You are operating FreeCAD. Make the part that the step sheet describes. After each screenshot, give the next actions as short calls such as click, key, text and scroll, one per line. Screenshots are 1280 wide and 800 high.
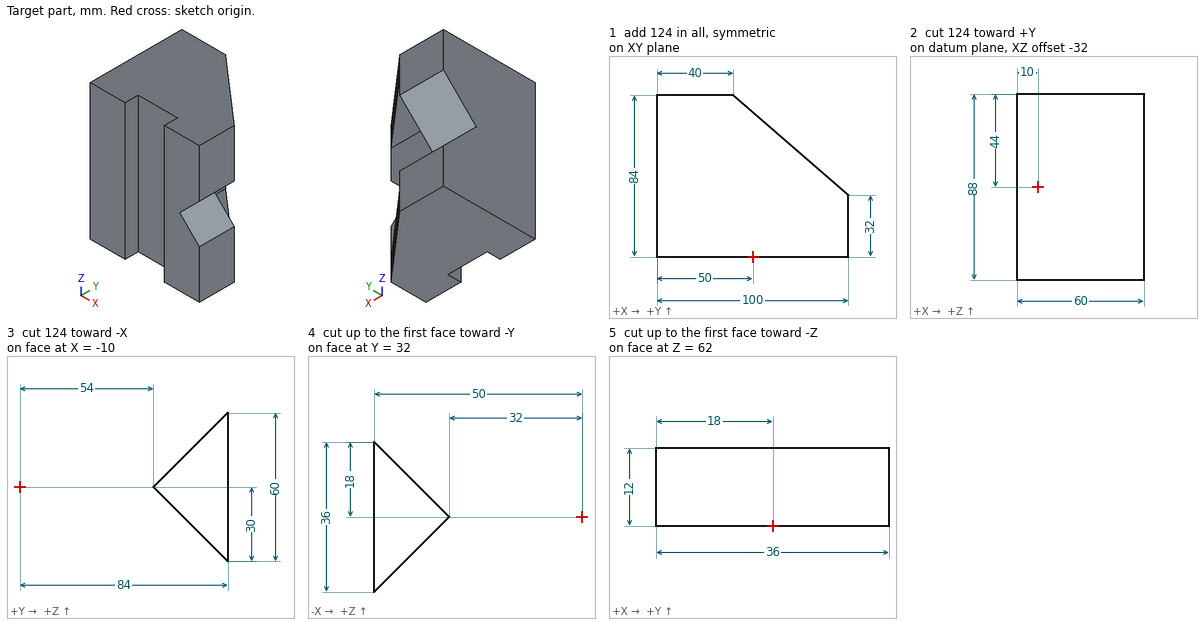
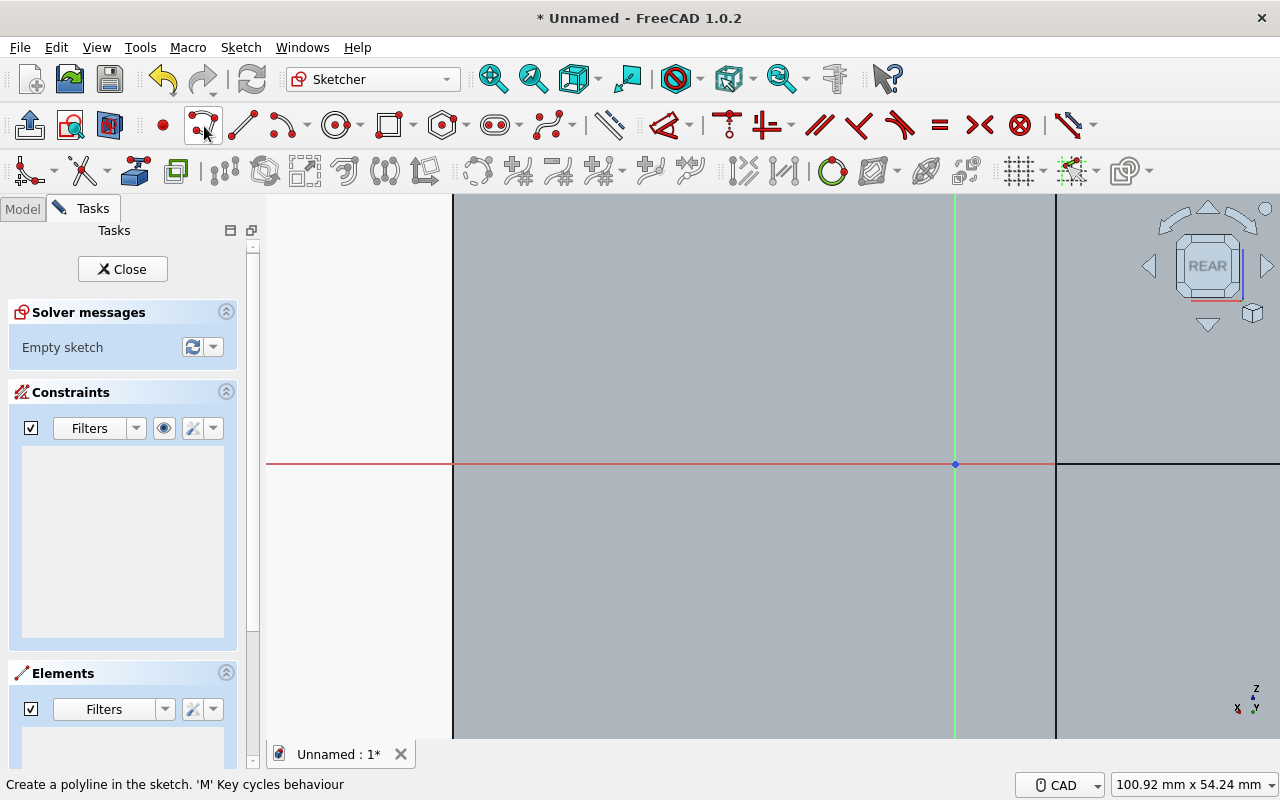
click(634, 464)
click(453, 283)
click(453, 645)
click(634, 464)
key(Escape)
key(Escape)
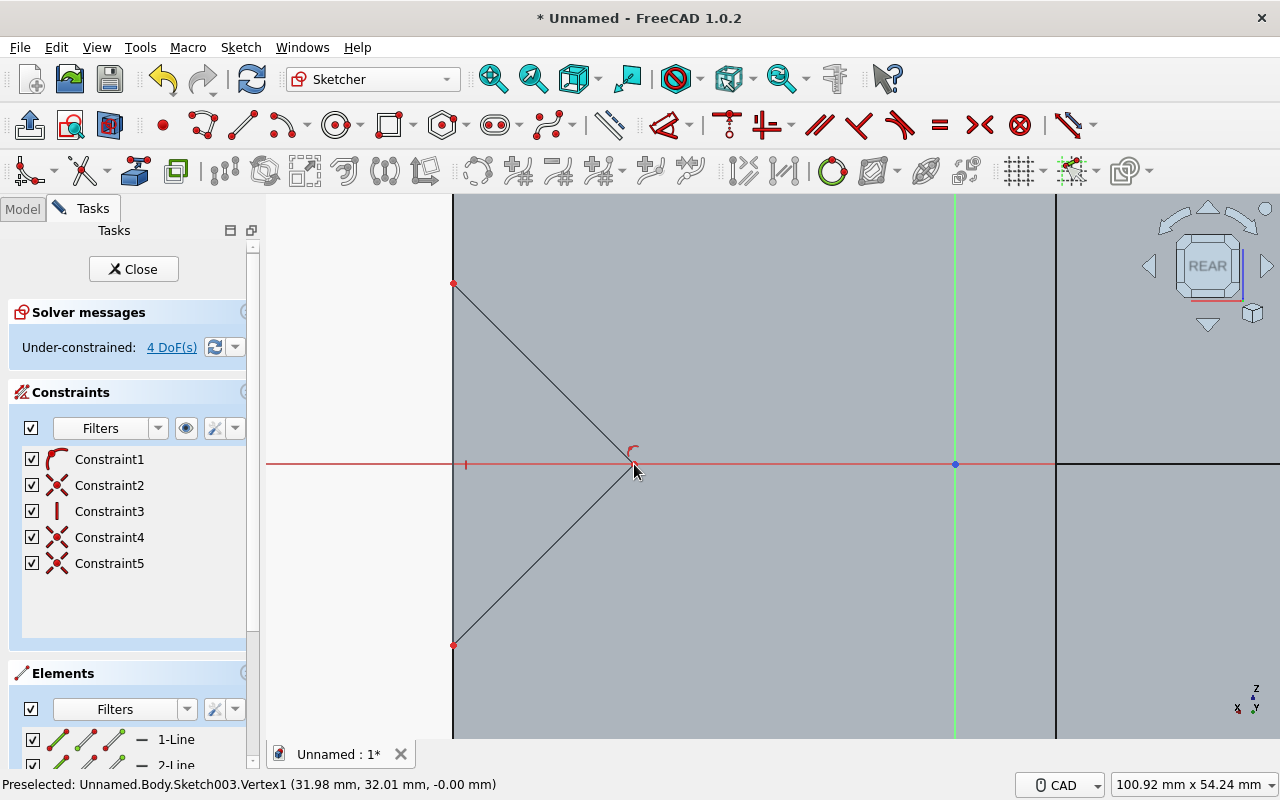
click(664, 126)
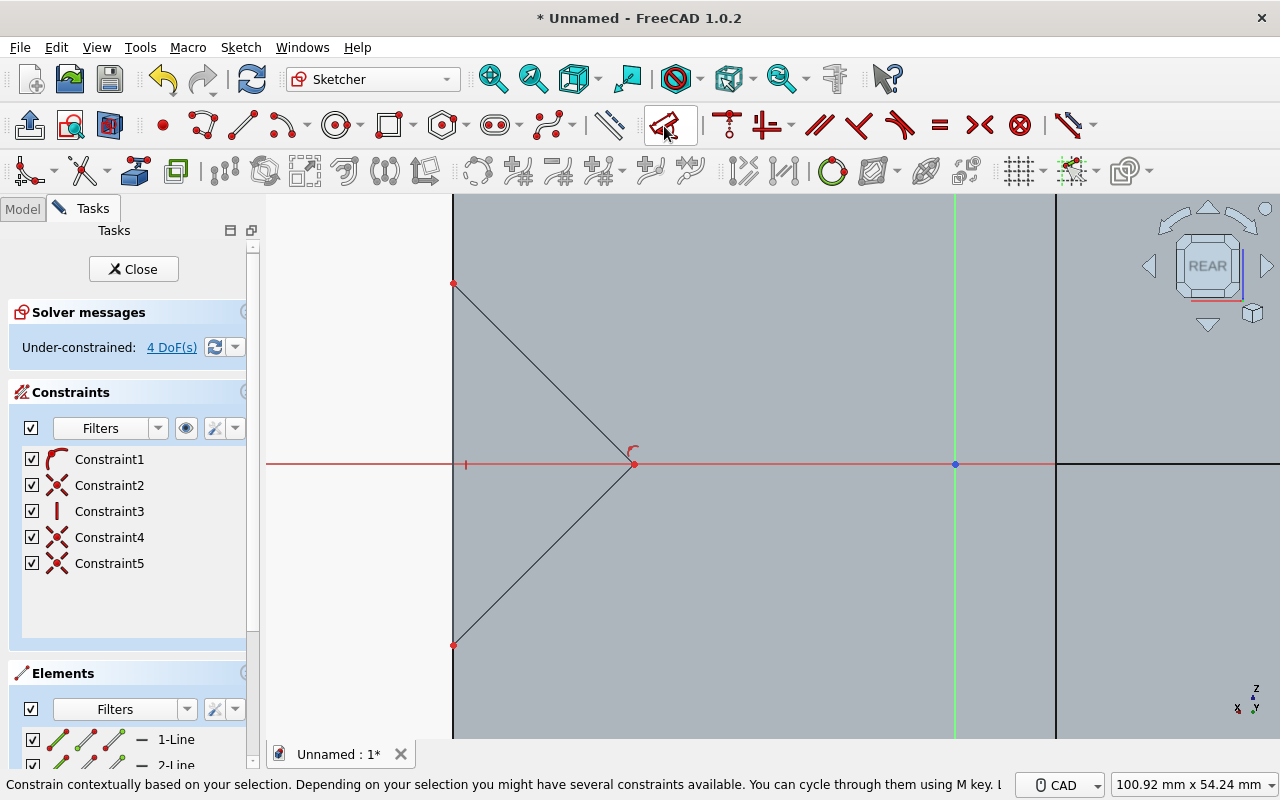
click(453, 393)
click(419, 382)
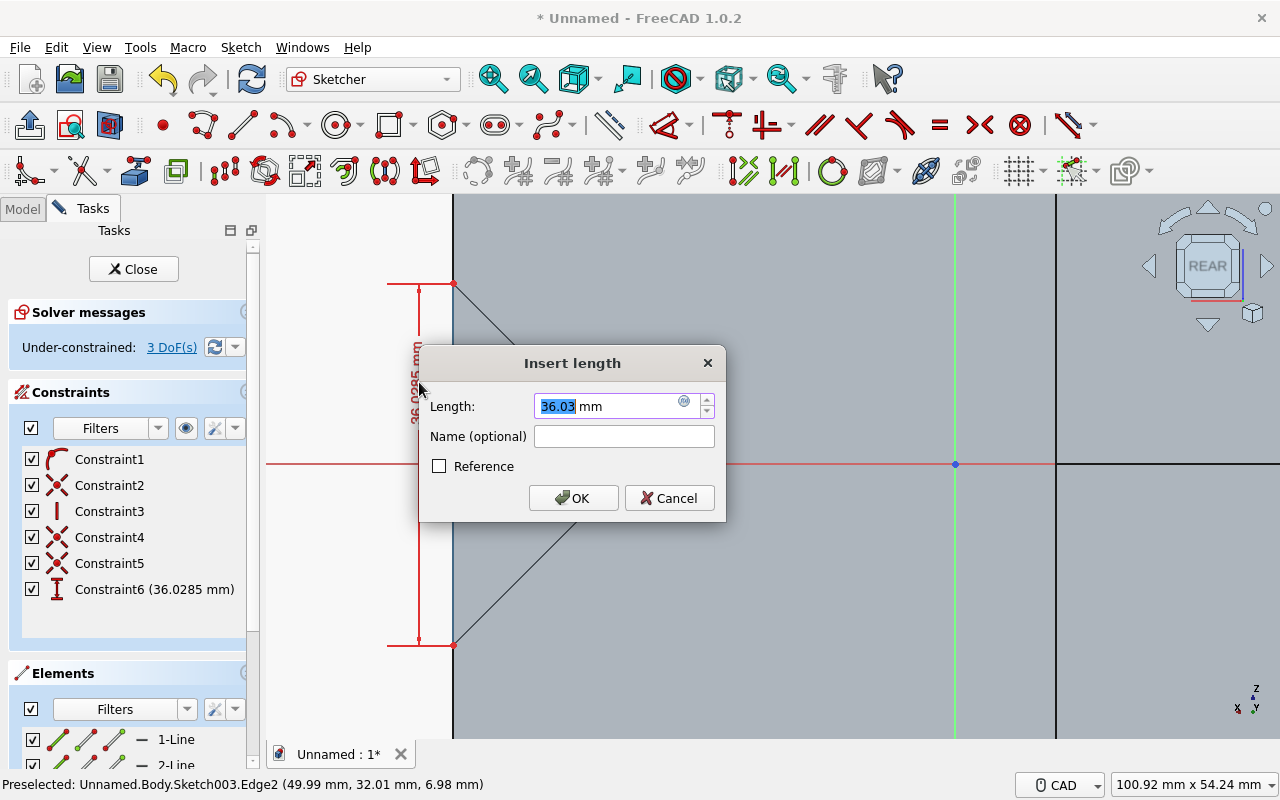
text(36)
key(Return)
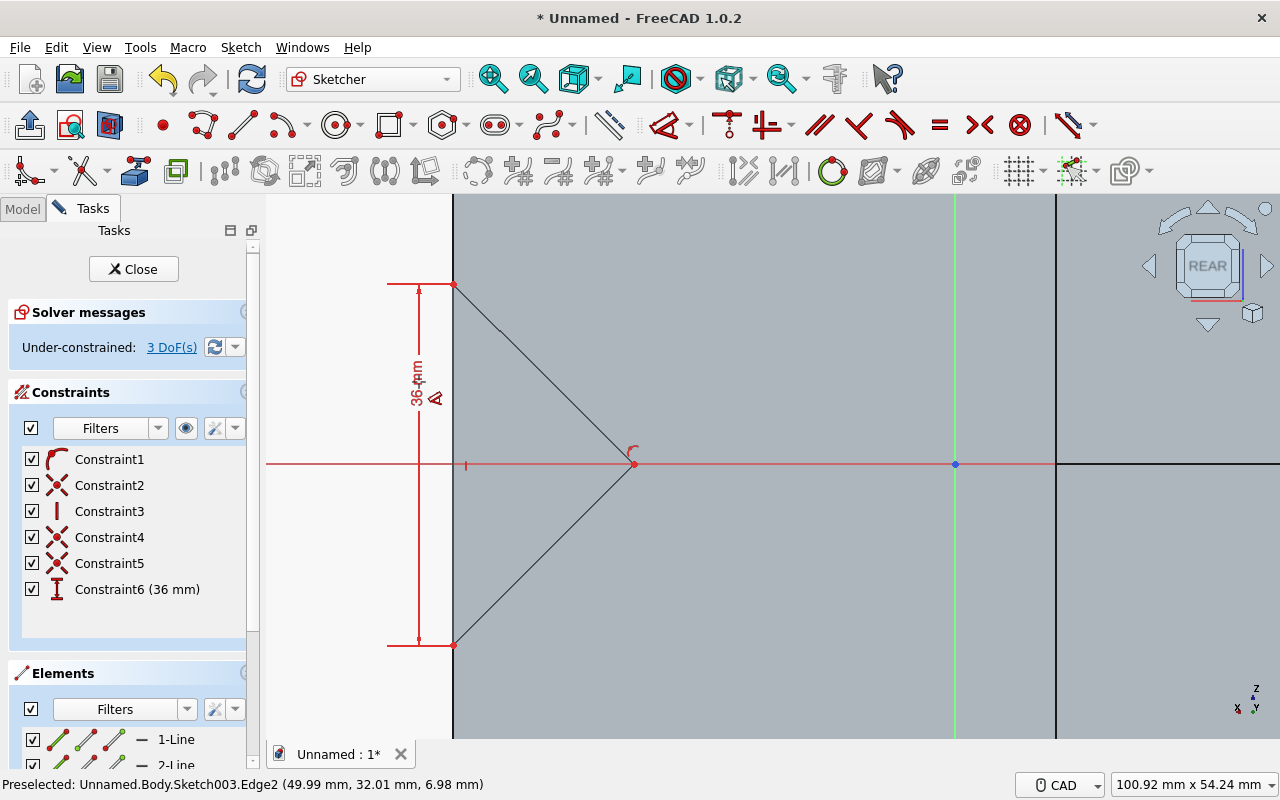
click(634, 464)
click(795, 498)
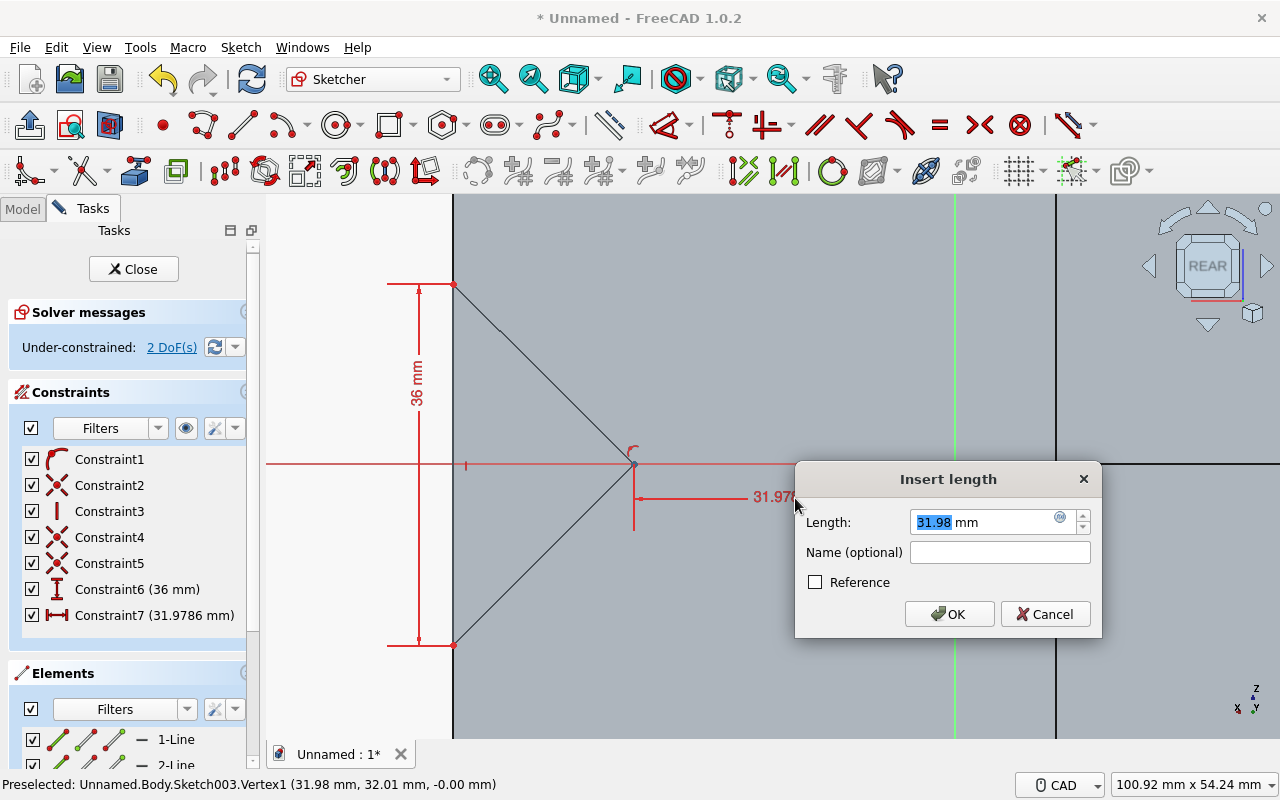
text(32)
key(Return)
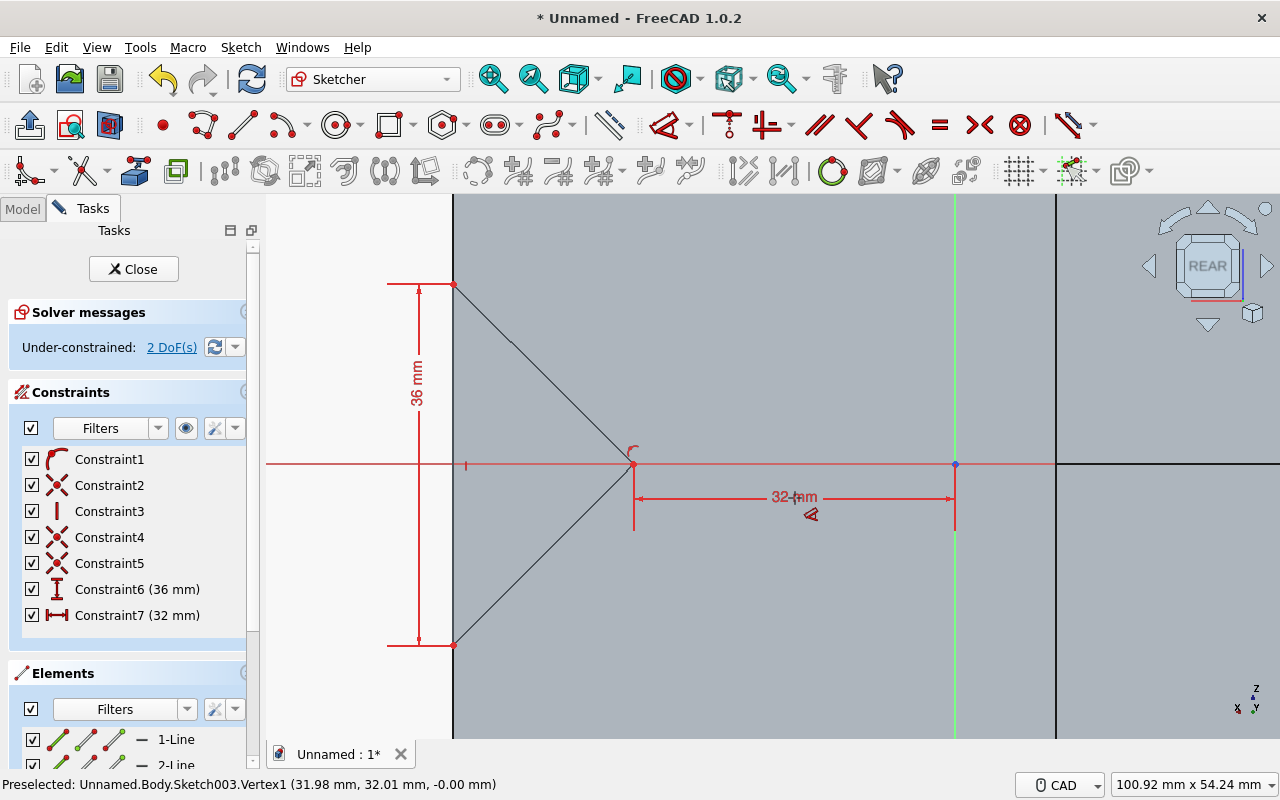
click(453, 284)
click(704, 250)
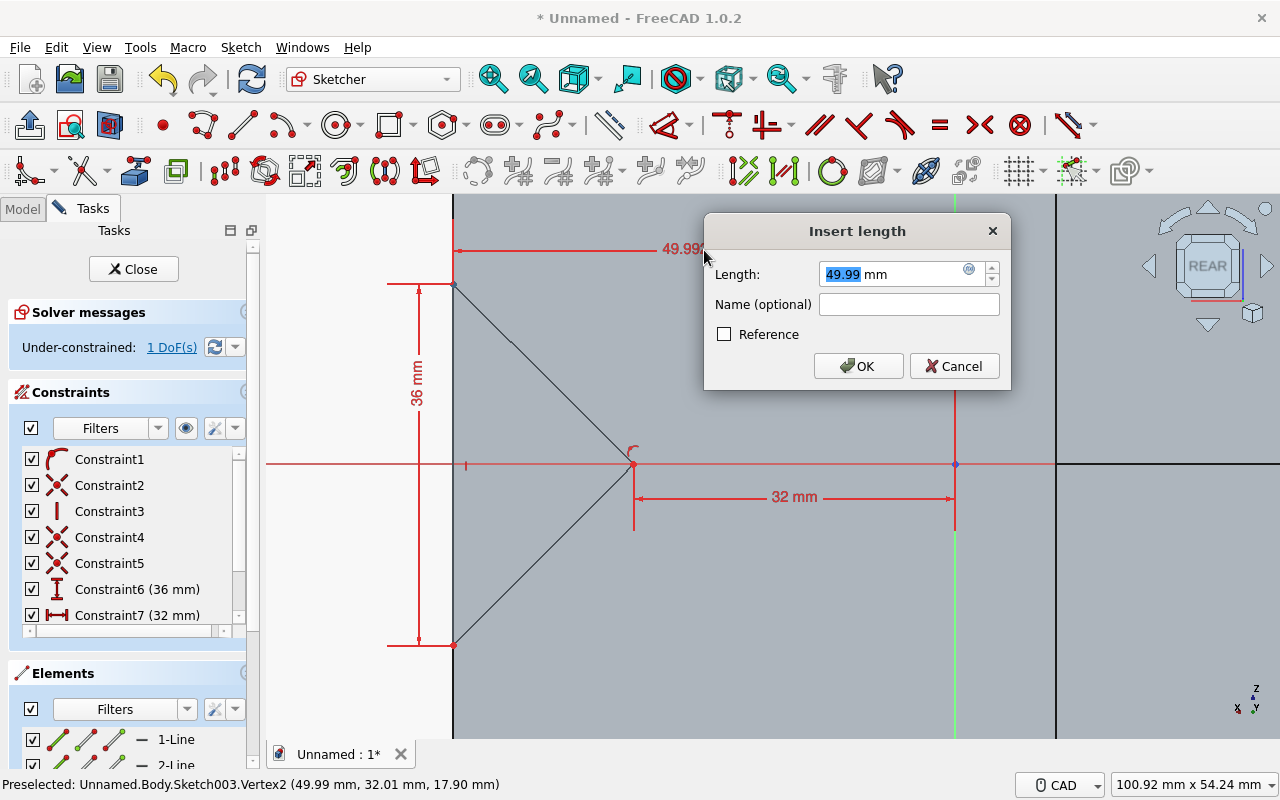
text(50)
key(Return)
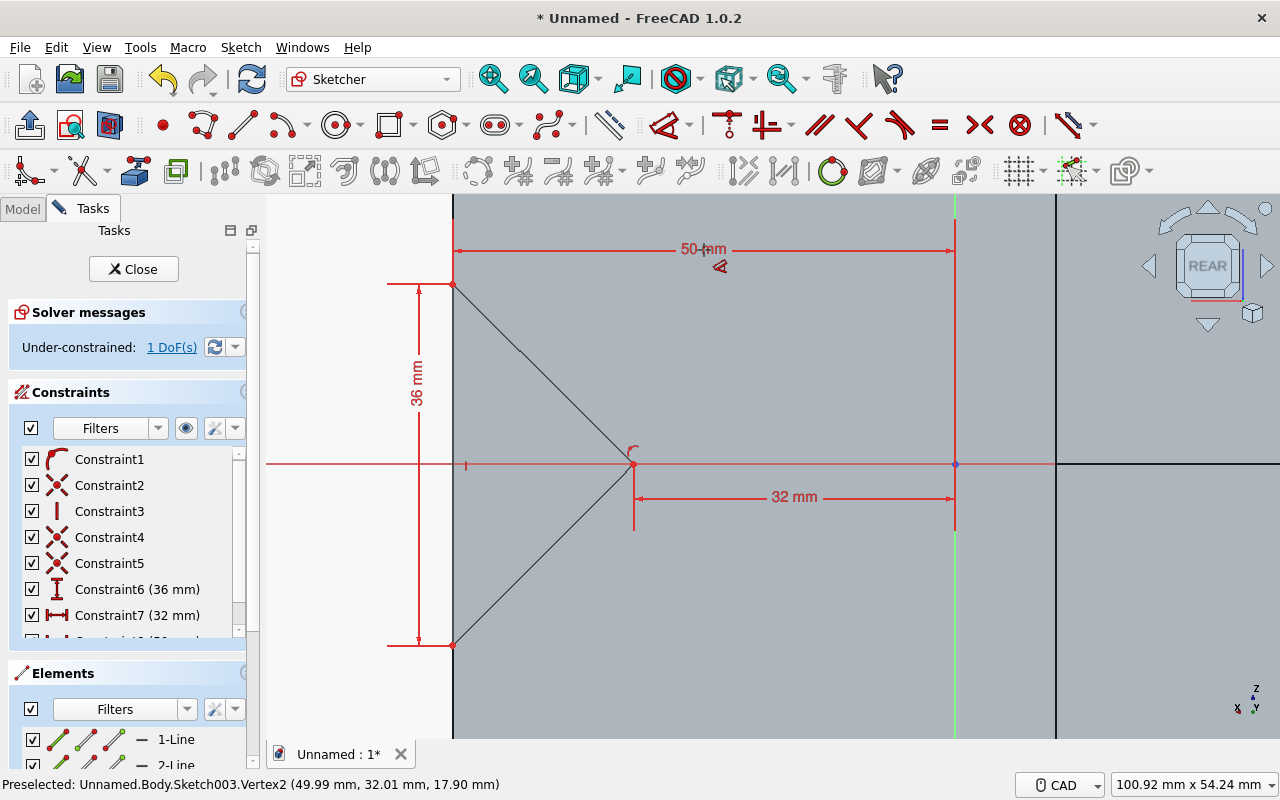
click(453, 284)
click(989, 374)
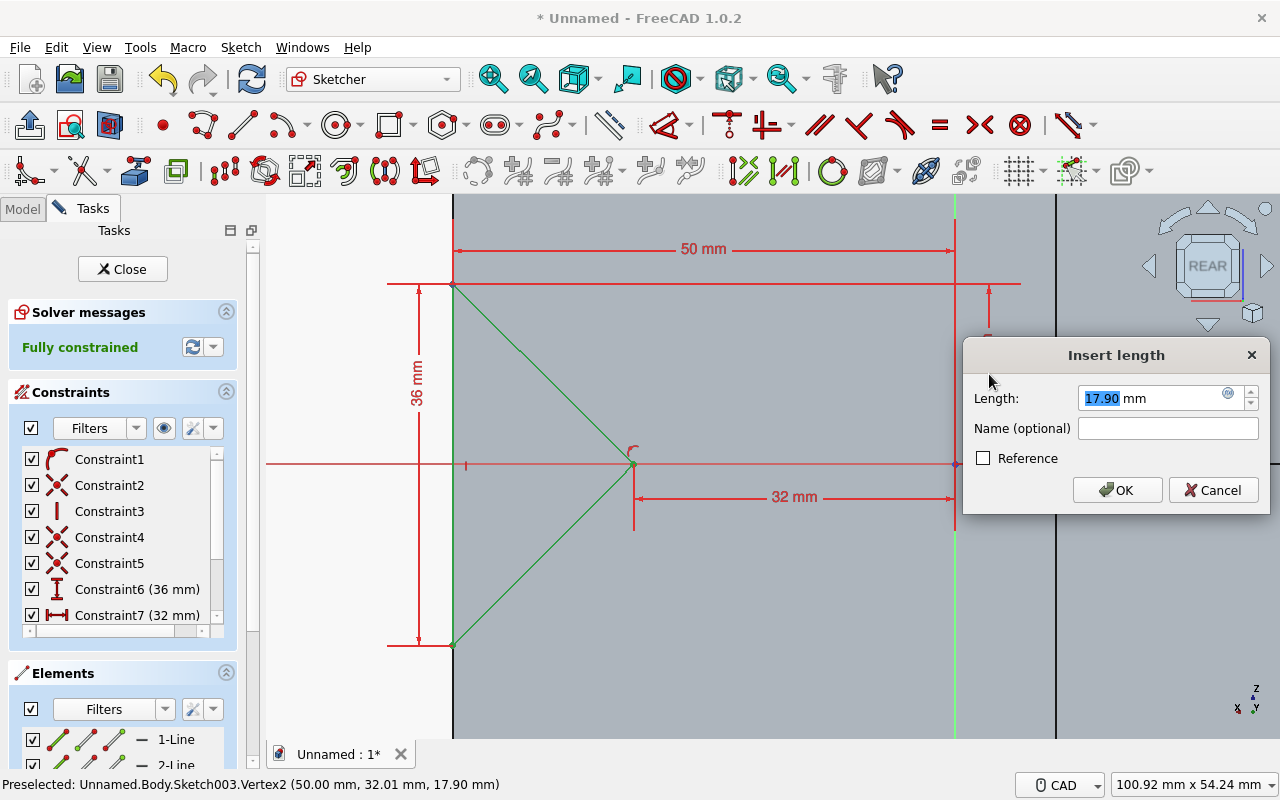
text(18)
key(Return)
key(Escape)